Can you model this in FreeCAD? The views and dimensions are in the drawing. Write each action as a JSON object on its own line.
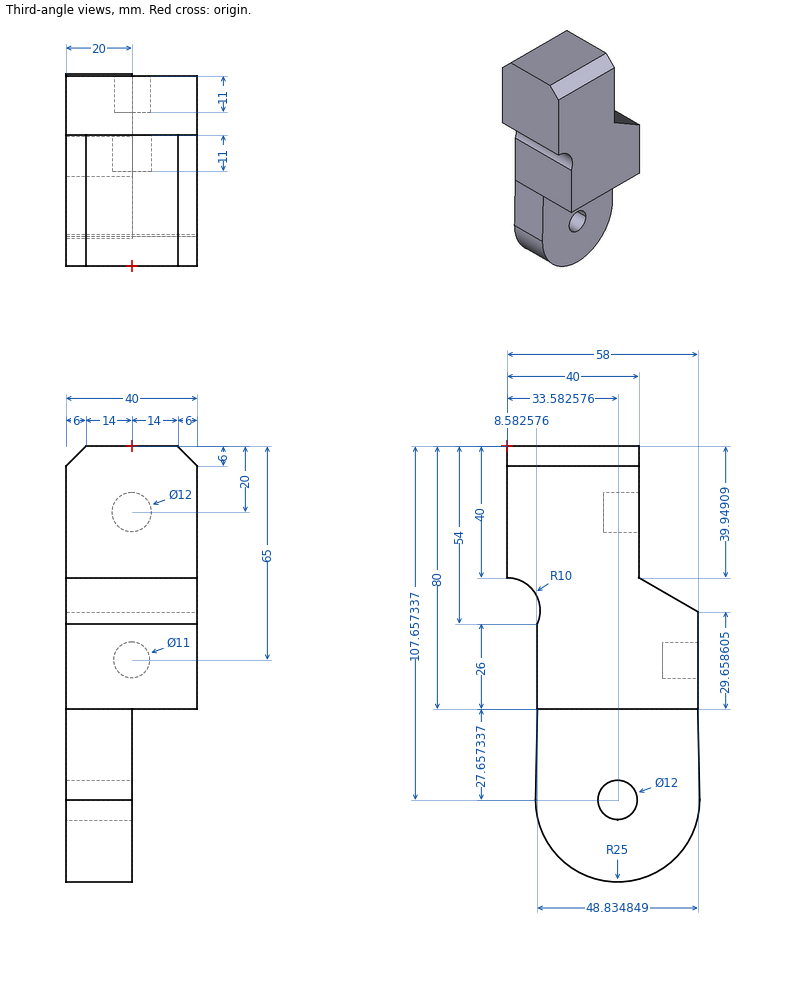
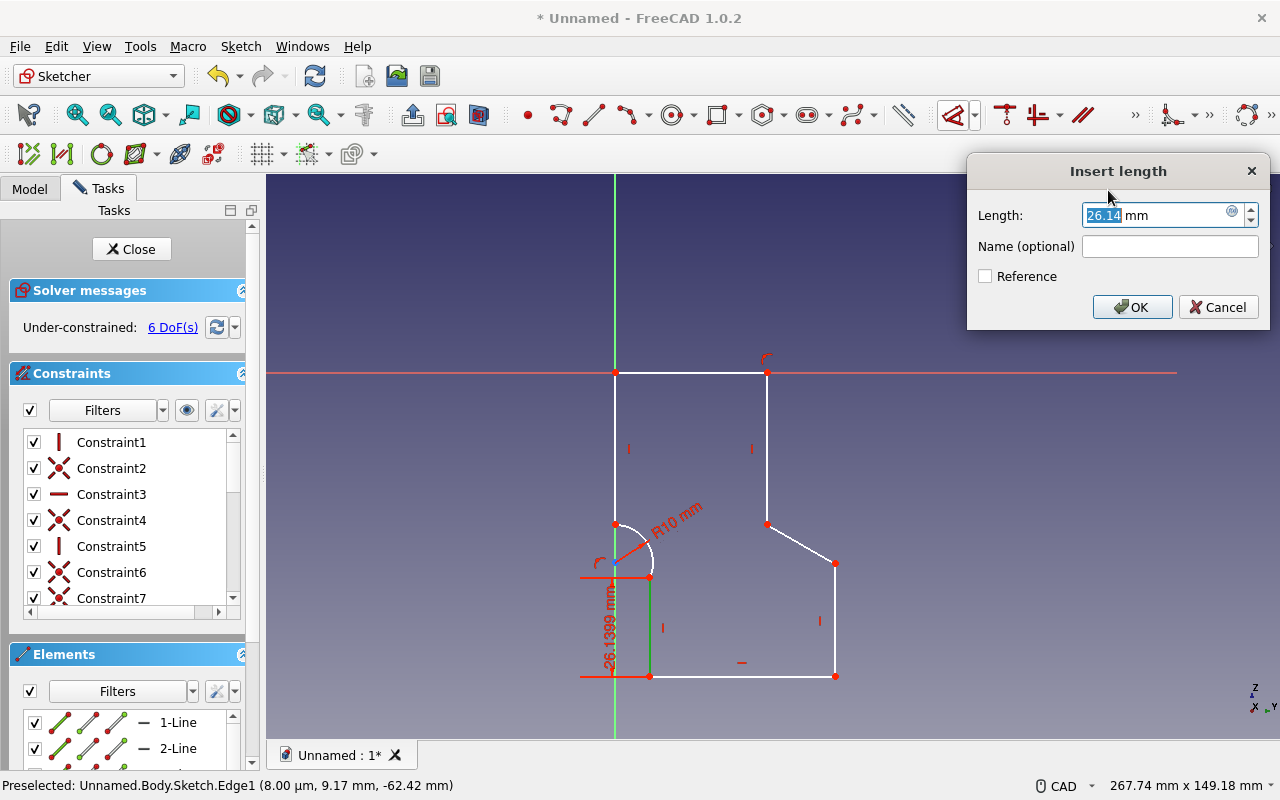
{"action": "type", "text": "26"}
{"action": "key", "text": "Return"}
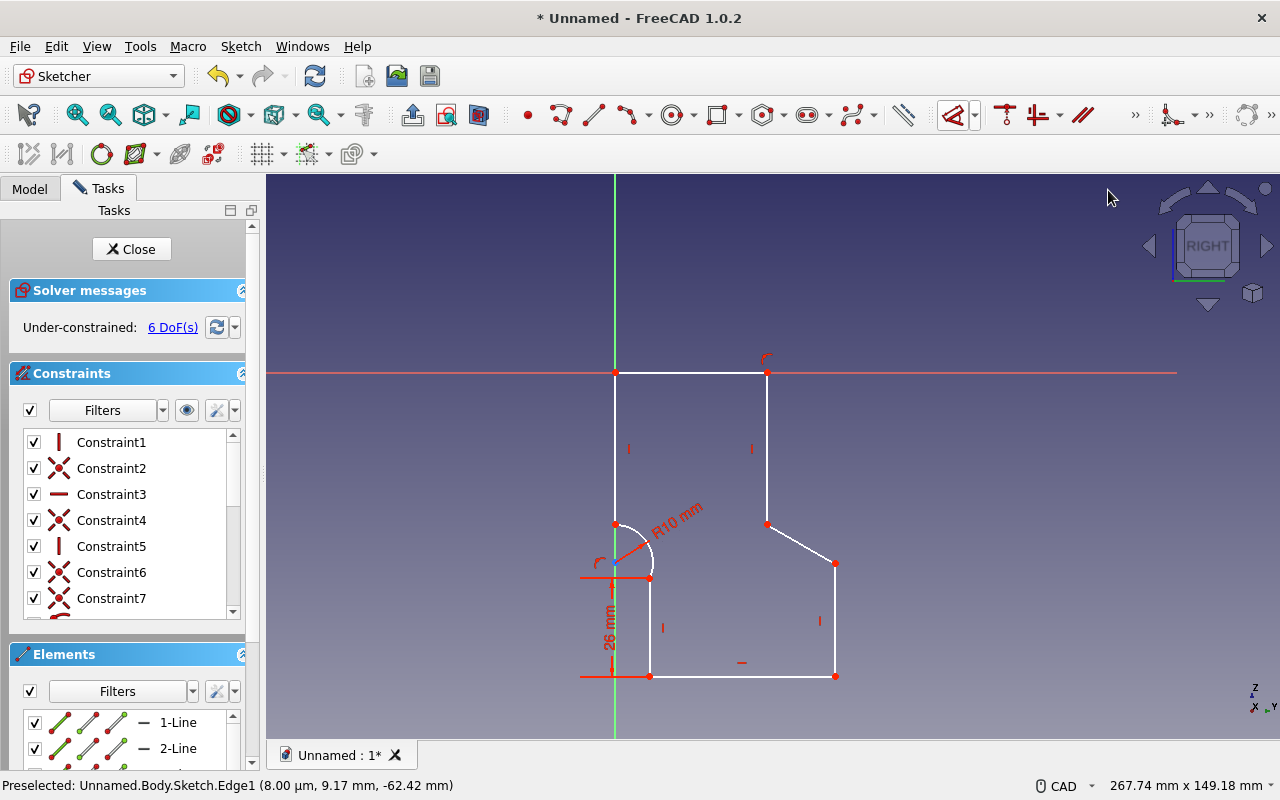
{"action": "left_click", "coordinate": [721, 373]}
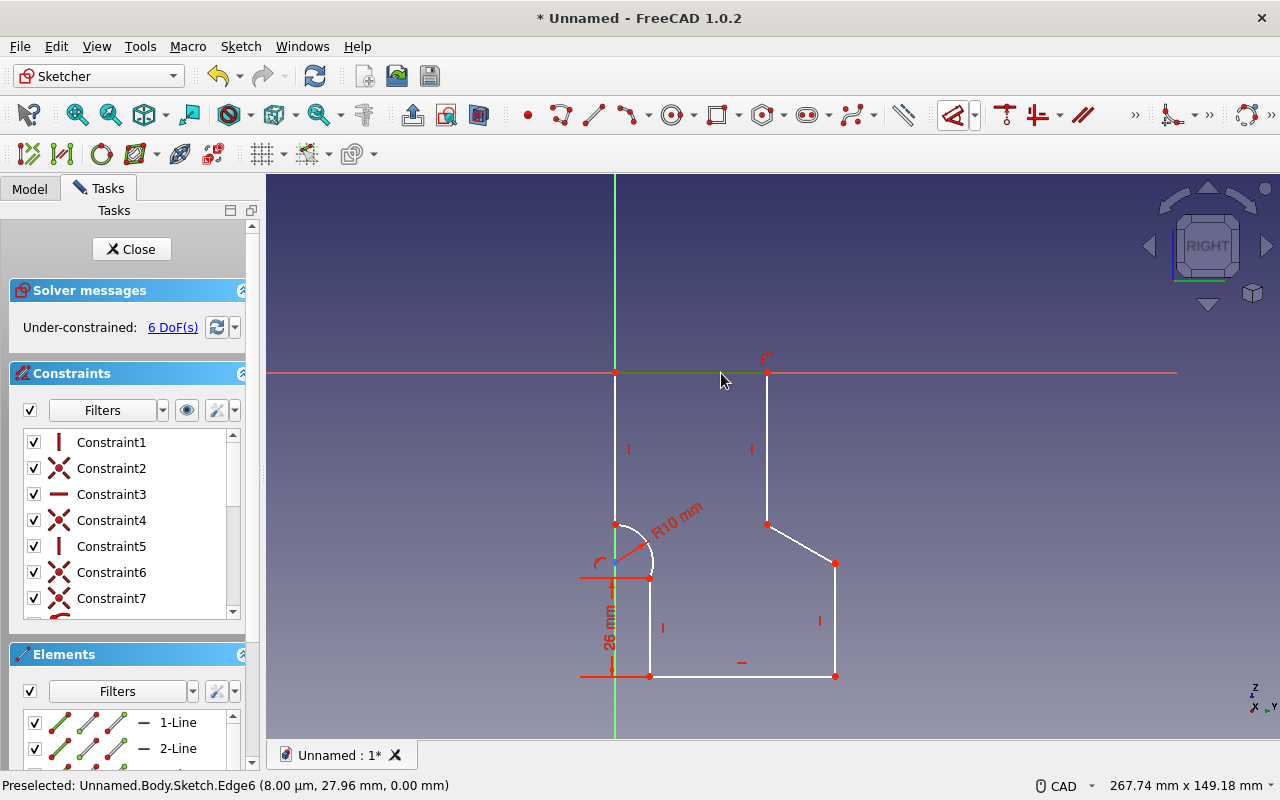
{"action": "left_click", "coordinate": [974, 116]}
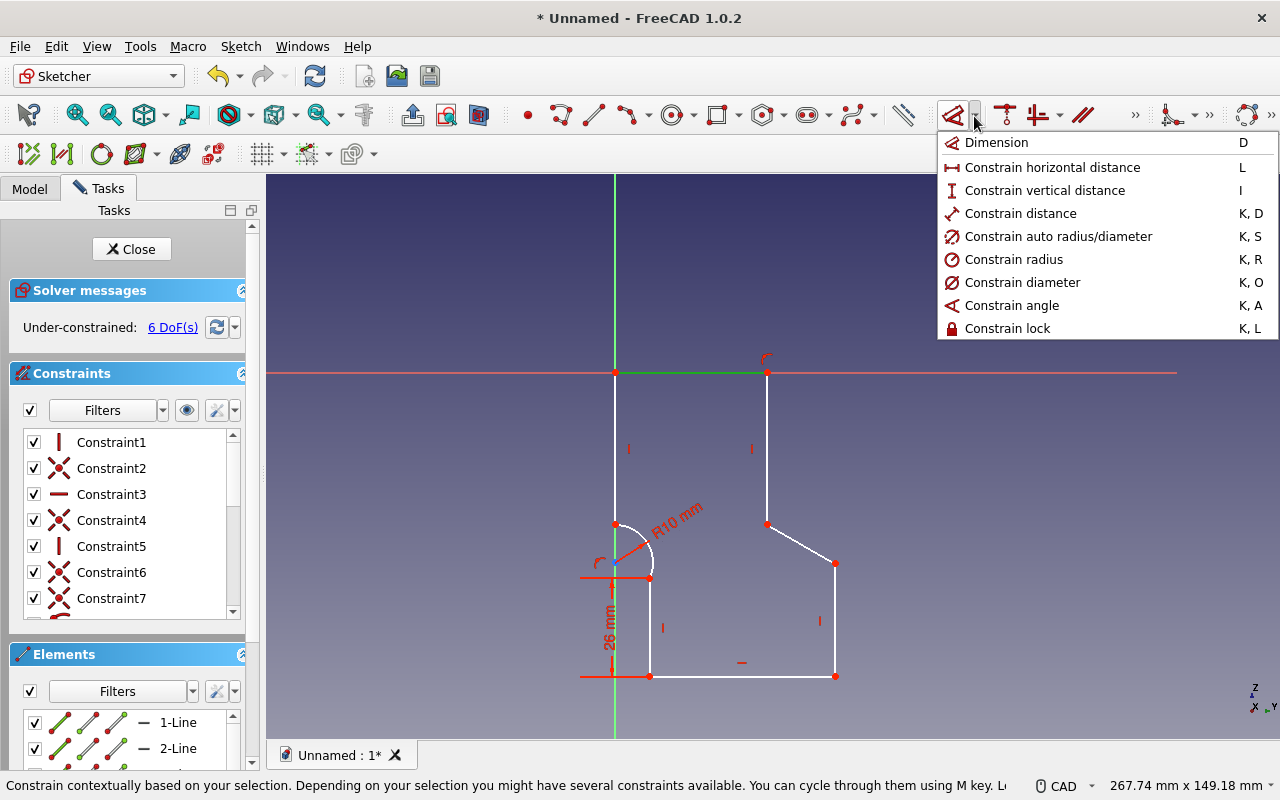
{"action": "left_click", "coordinate": [1108, 168]}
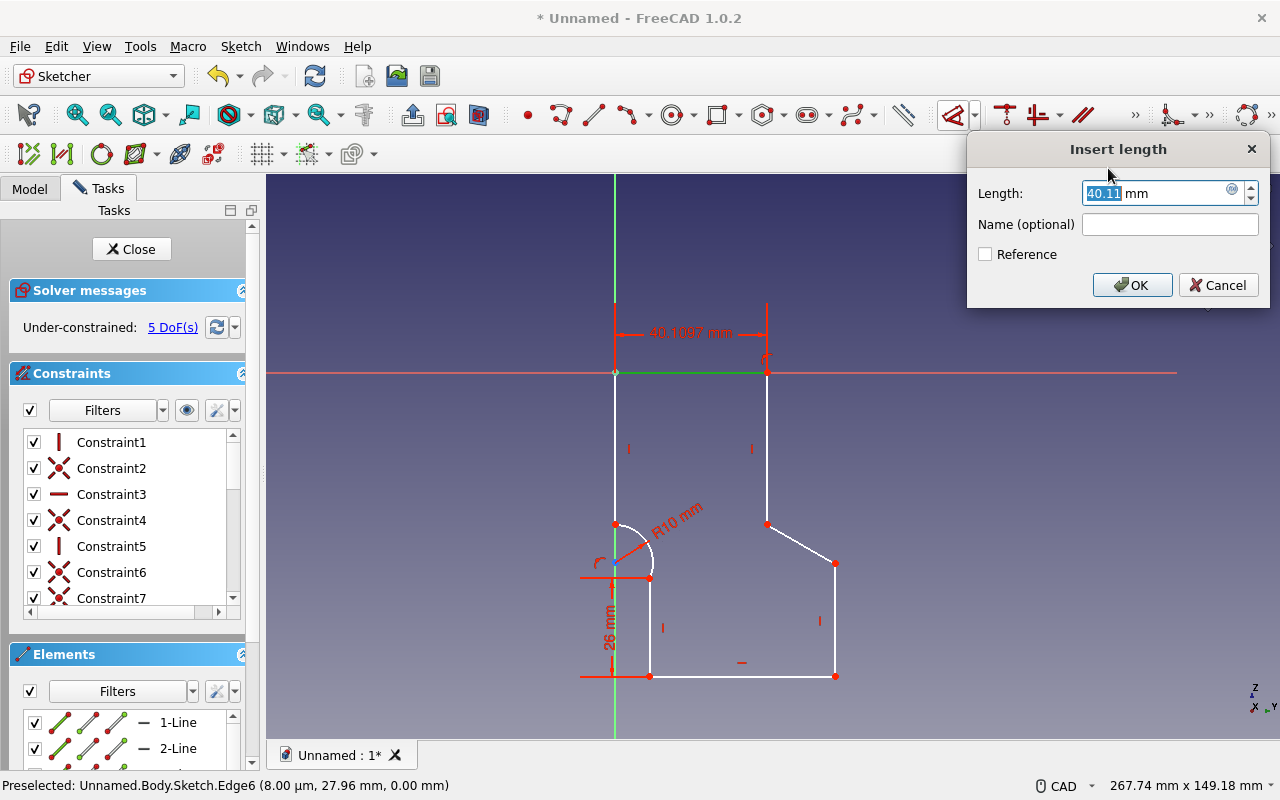
{"action": "type", "text": "40"}
{"action": "key", "text": "Return"}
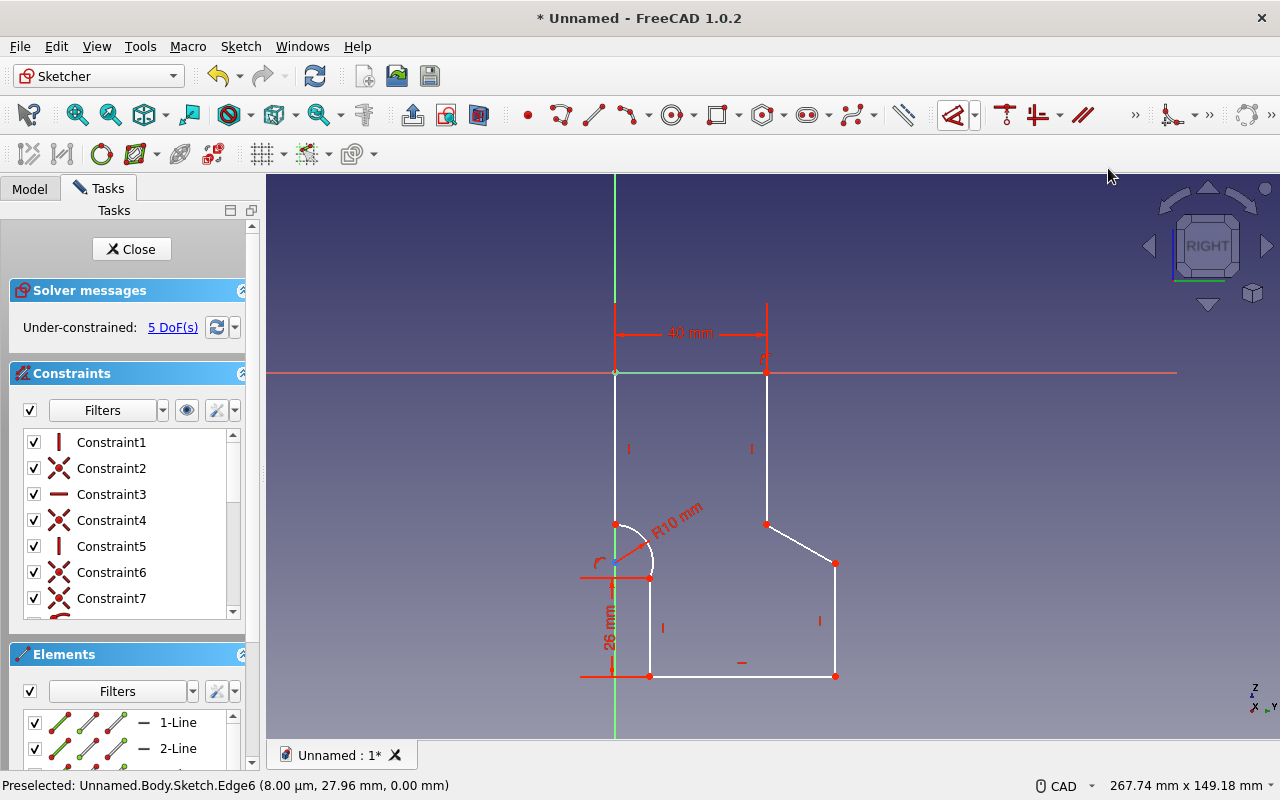
{"action": "left_click", "coordinate": [615, 418]}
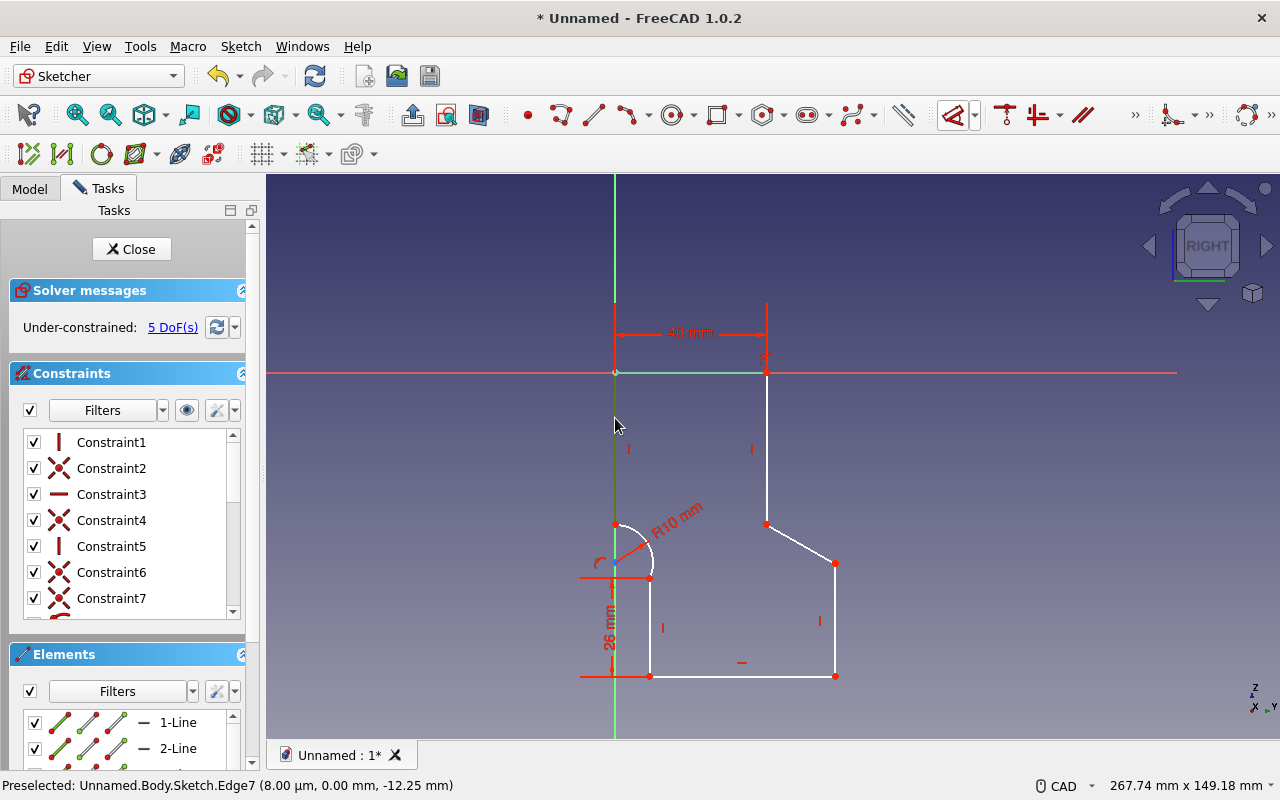
{"action": "key", "text": "i"}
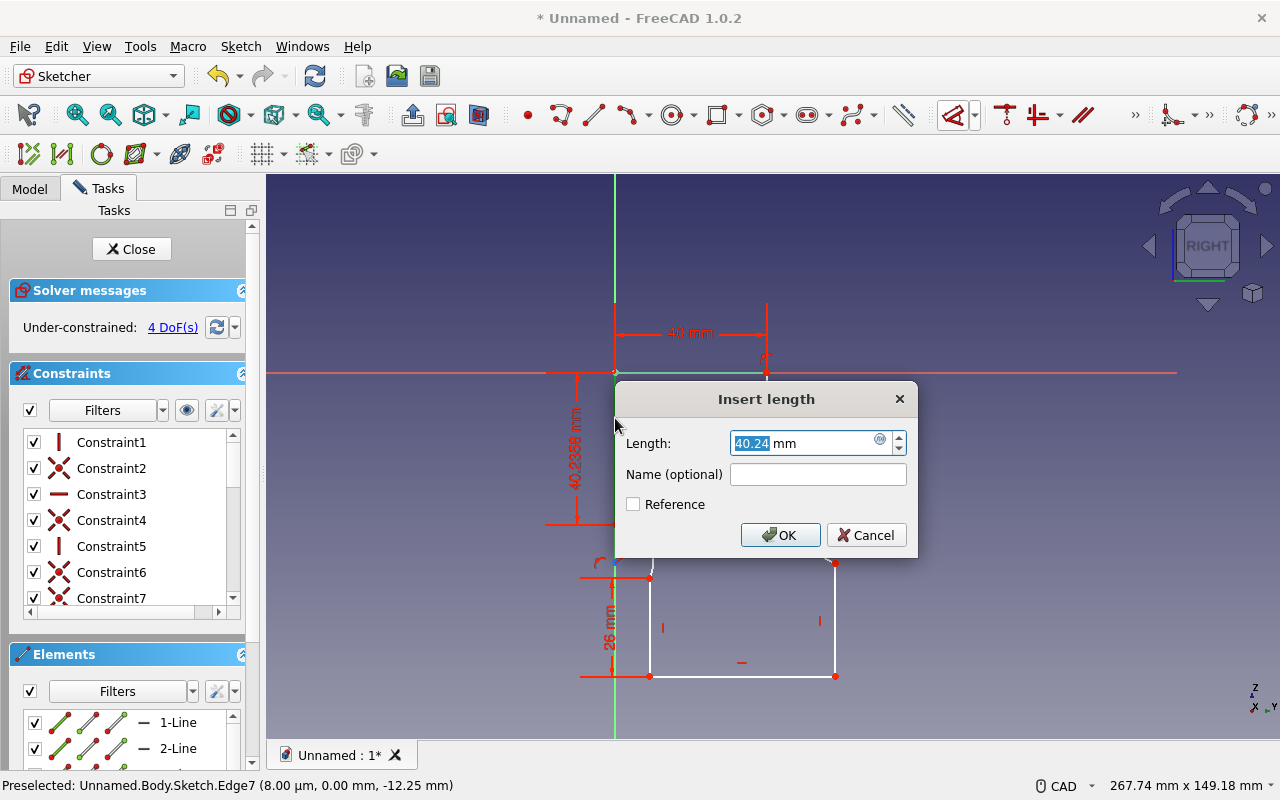
{"action": "type", "text": "40"}
{"action": "key", "text": "Return"}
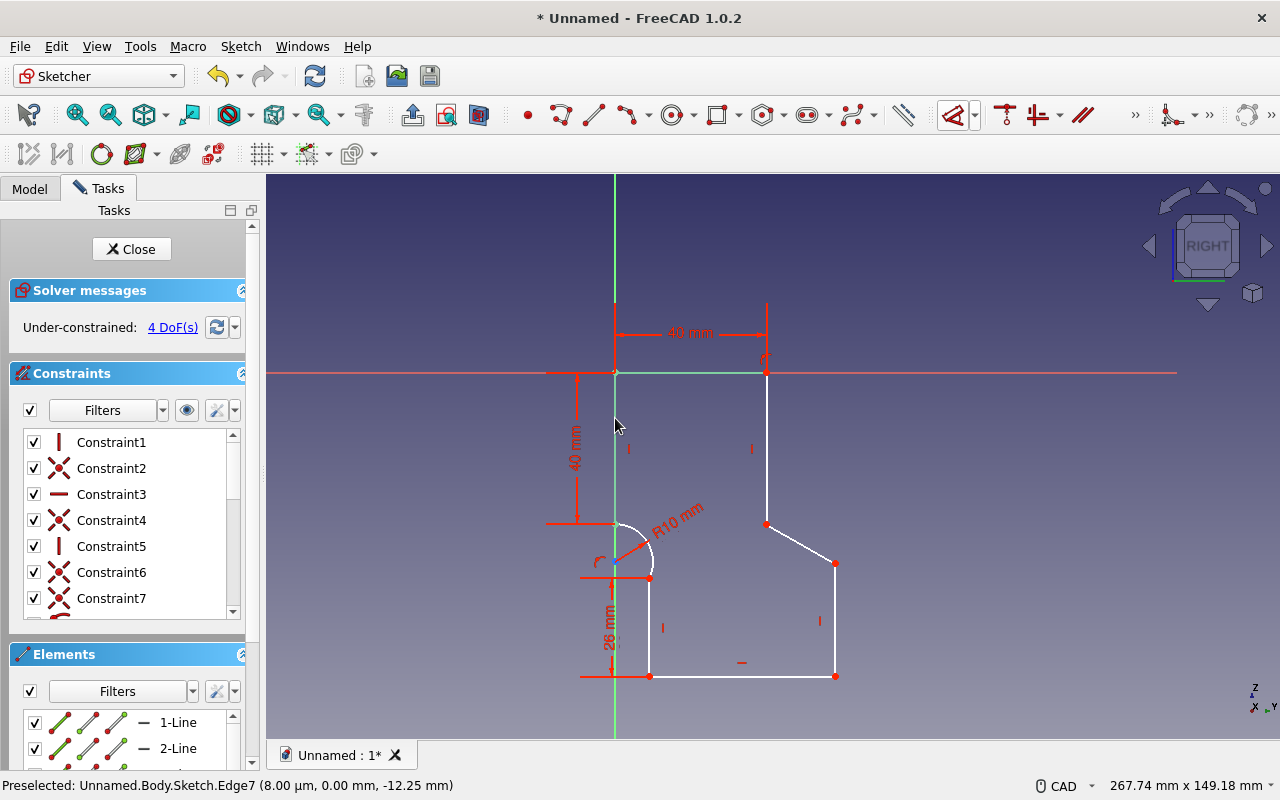
{"action": "left_click", "coordinate": [649, 578]}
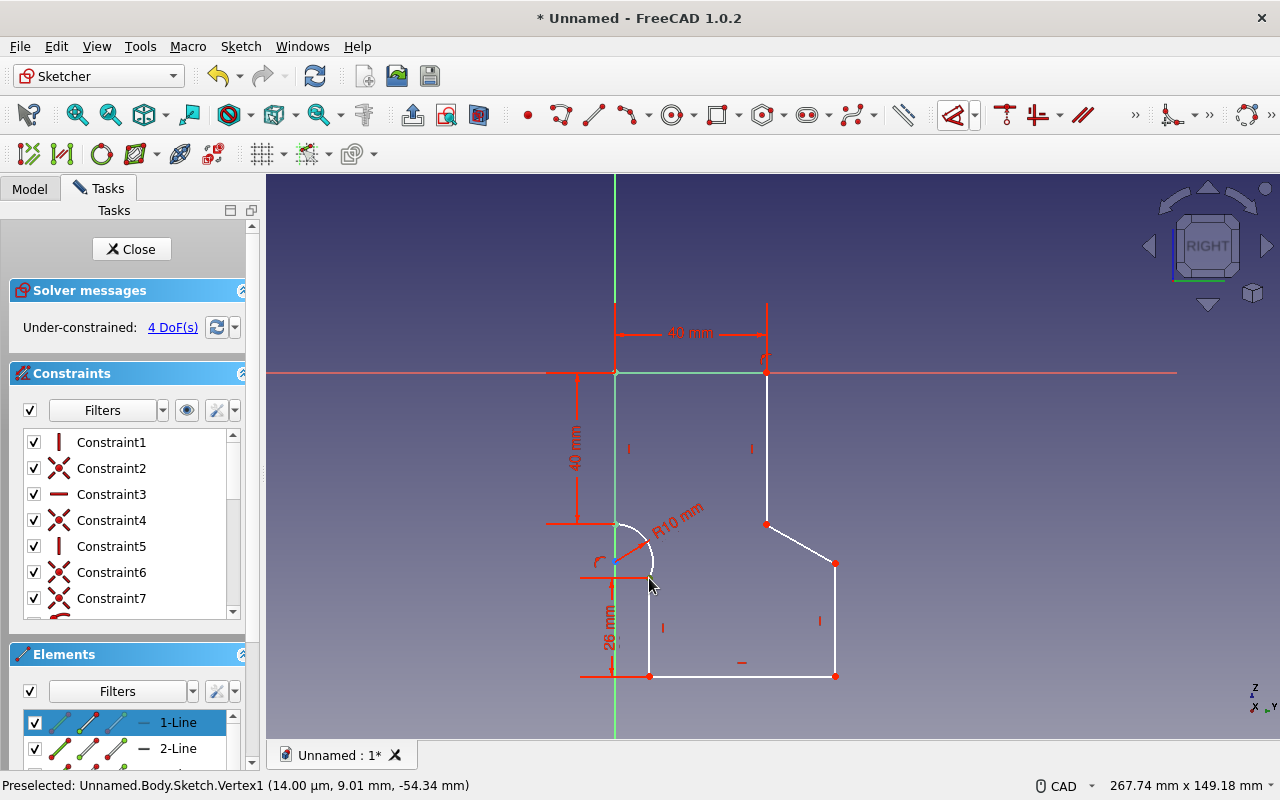
{"action": "key", "text": "i"}